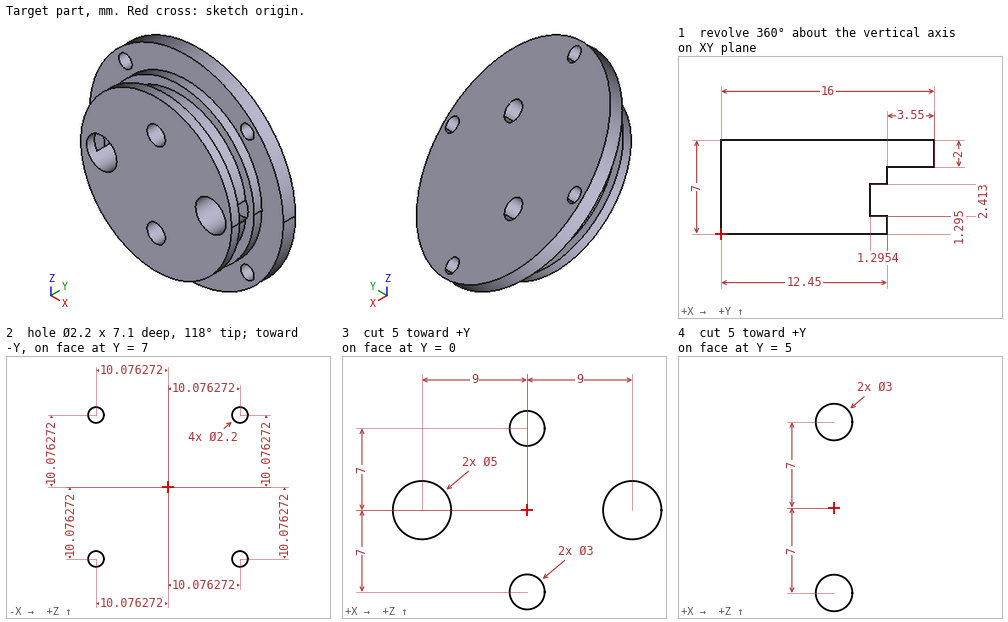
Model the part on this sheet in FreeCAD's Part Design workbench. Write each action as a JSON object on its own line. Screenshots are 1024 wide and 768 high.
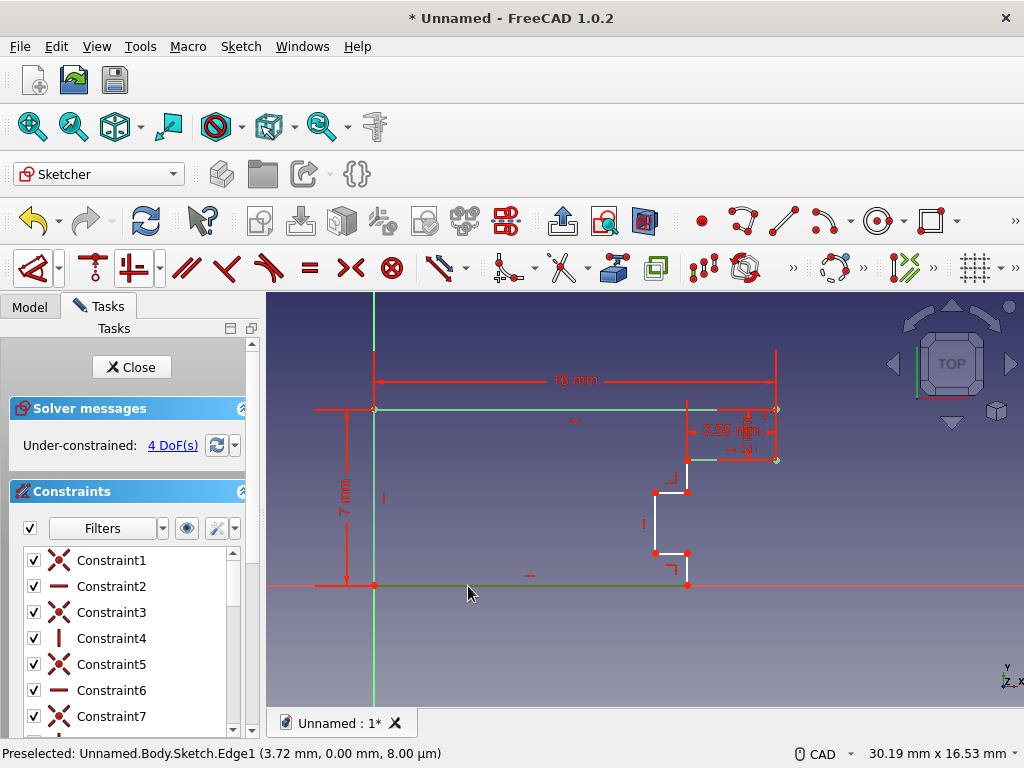
{"action": "left_click", "coordinate": [58, 268]}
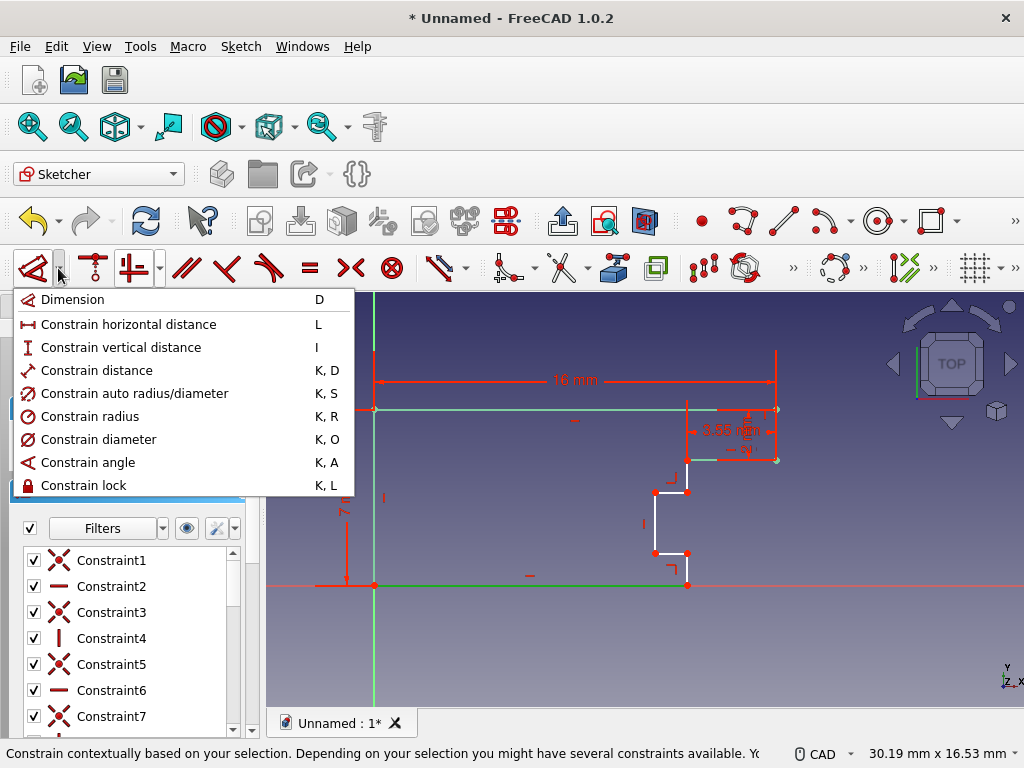
{"action": "left_click", "coordinate": [184, 324]}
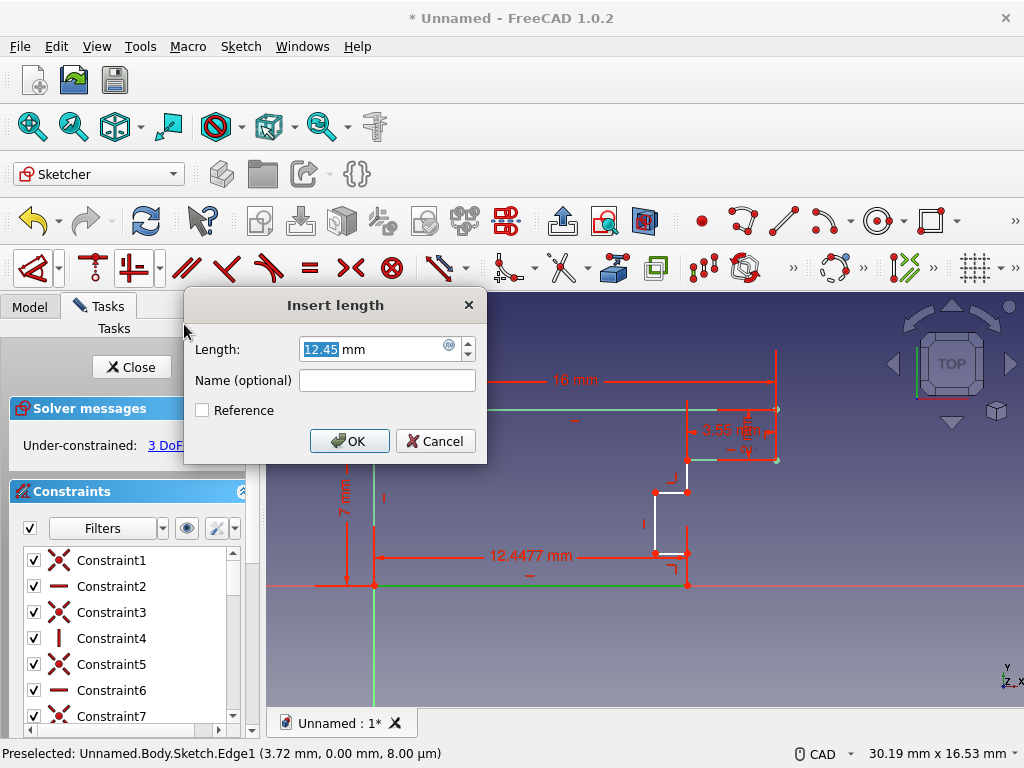
{"action": "type", "text": "12.45"}
{"action": "key", "text": "Return"}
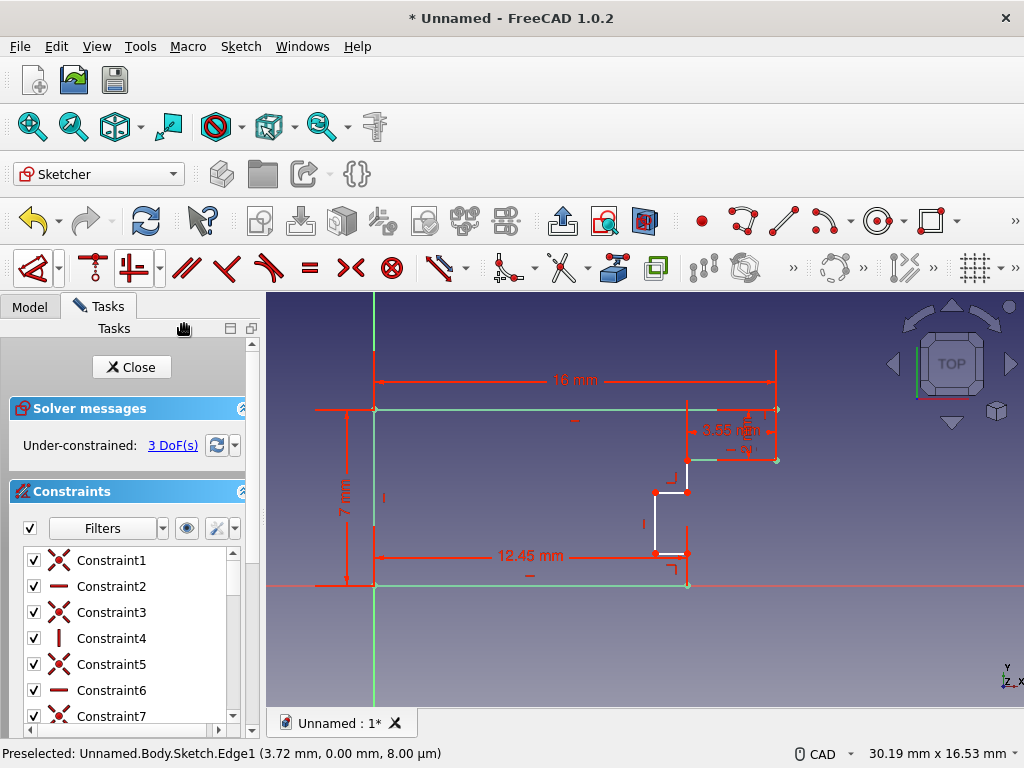
{"action": "scroll", "coordinate": [687, 576], "scroll_direction": "up", "scroll_amount": 2}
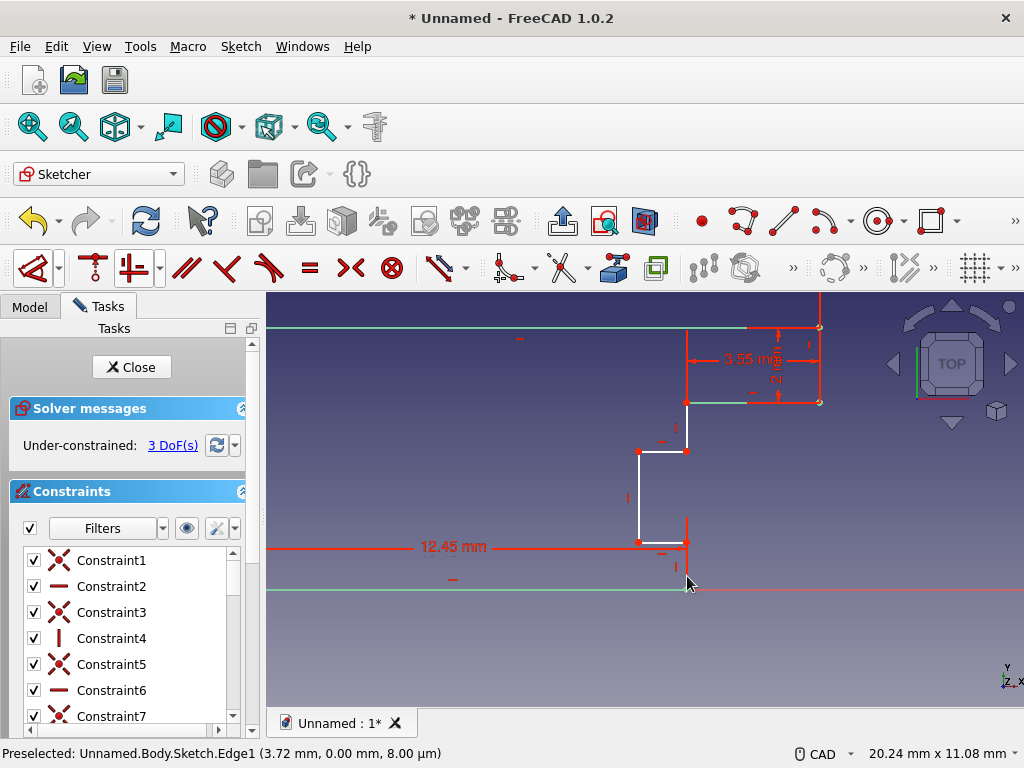
{"action": "left_click", "coordinate": [687, 576]}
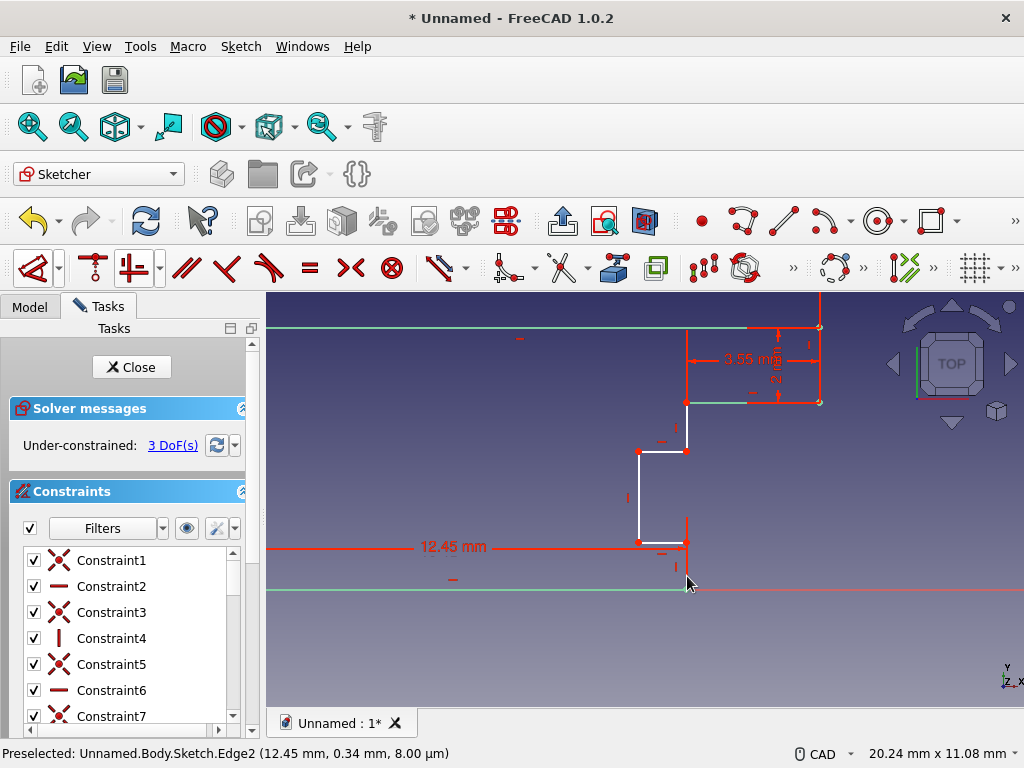
{"action": "key", "text": "i"}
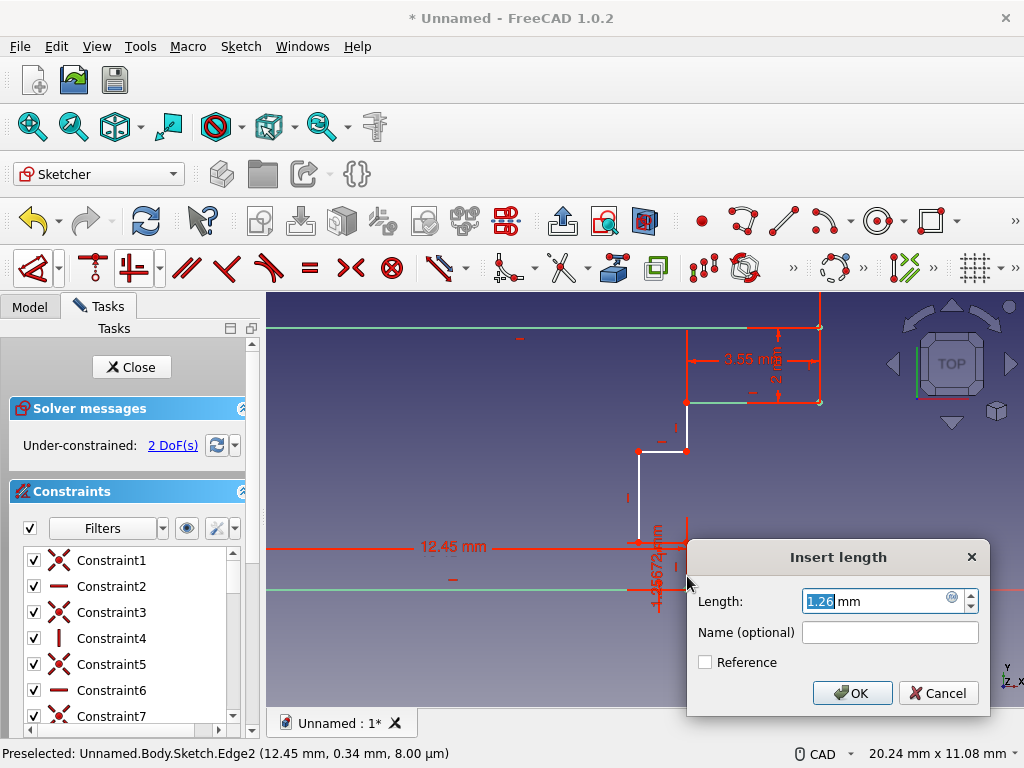
{"action": "type", "text": "1.295"}
{"action": "key", "text": "Return"}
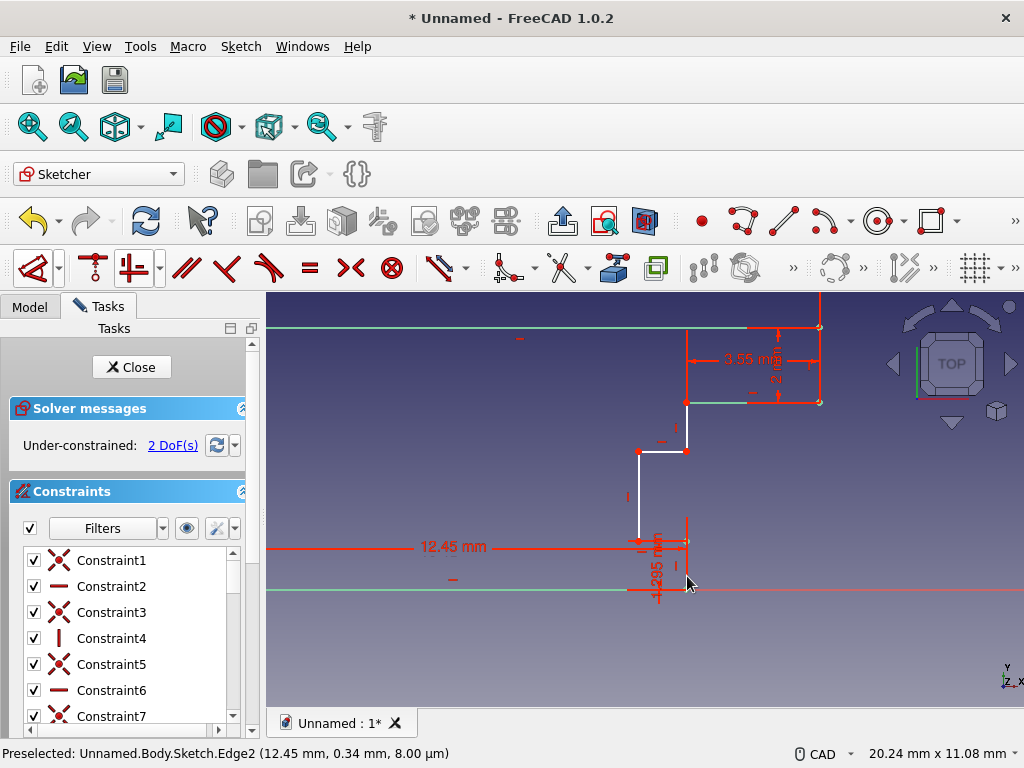
{"action": "left_click", "coordinate": [639, 515]}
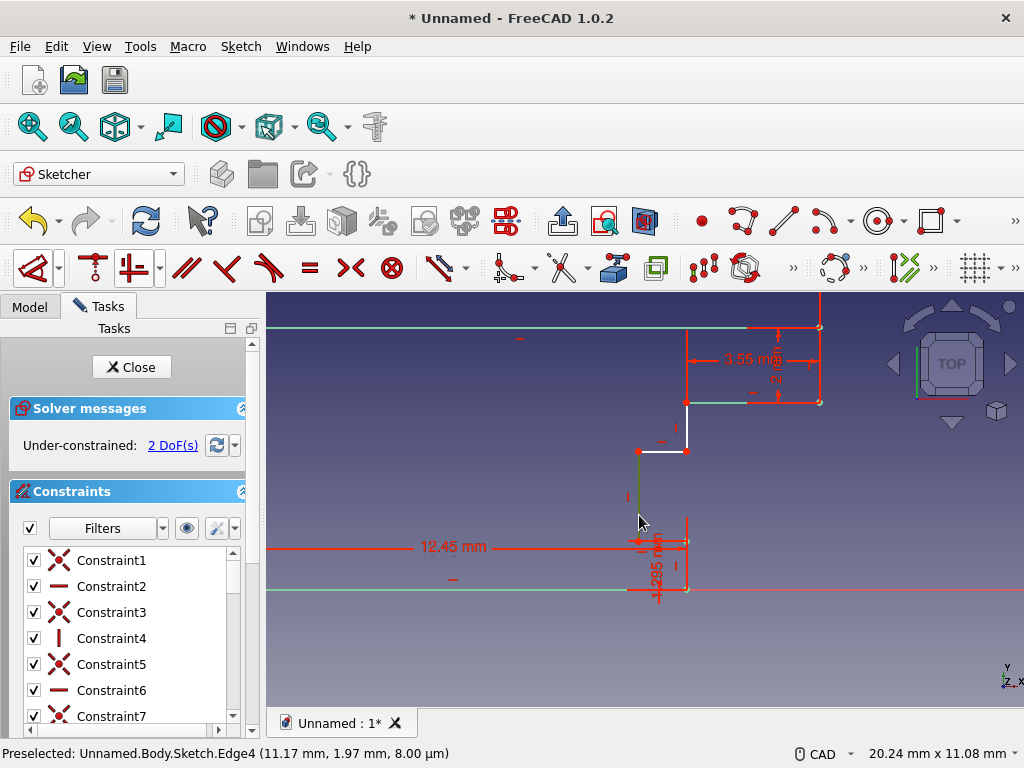
{"action": "key", "text": "i"}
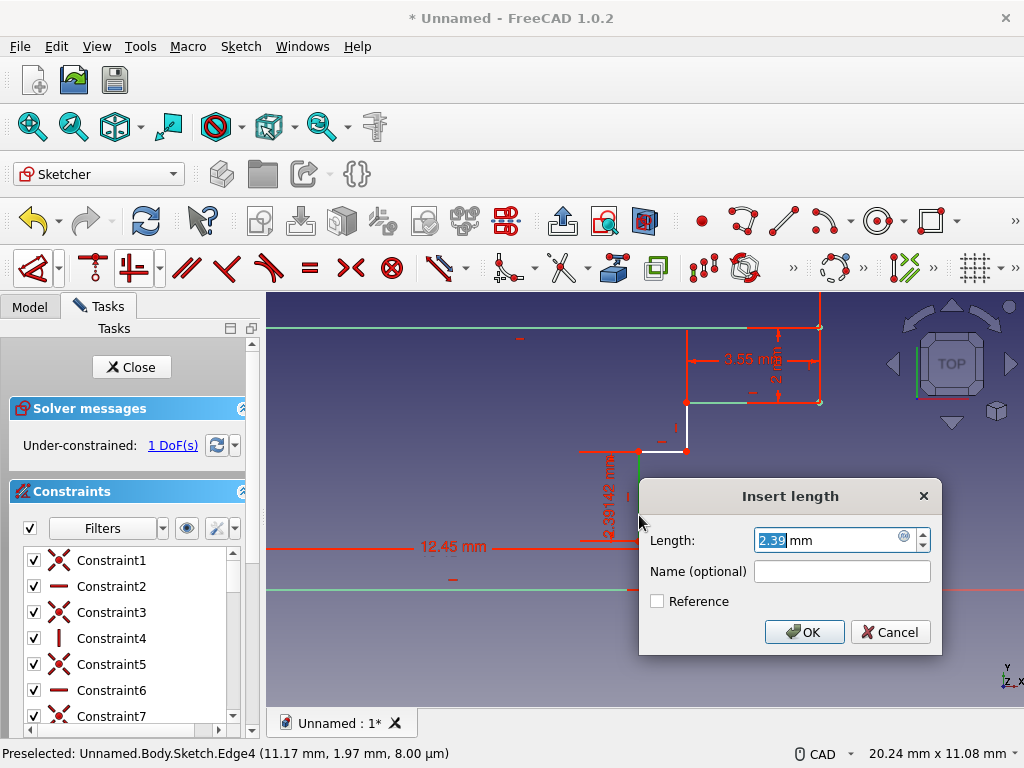
{"action": "type", "text": "2.413"}
{"action": "key", "text": "Return"}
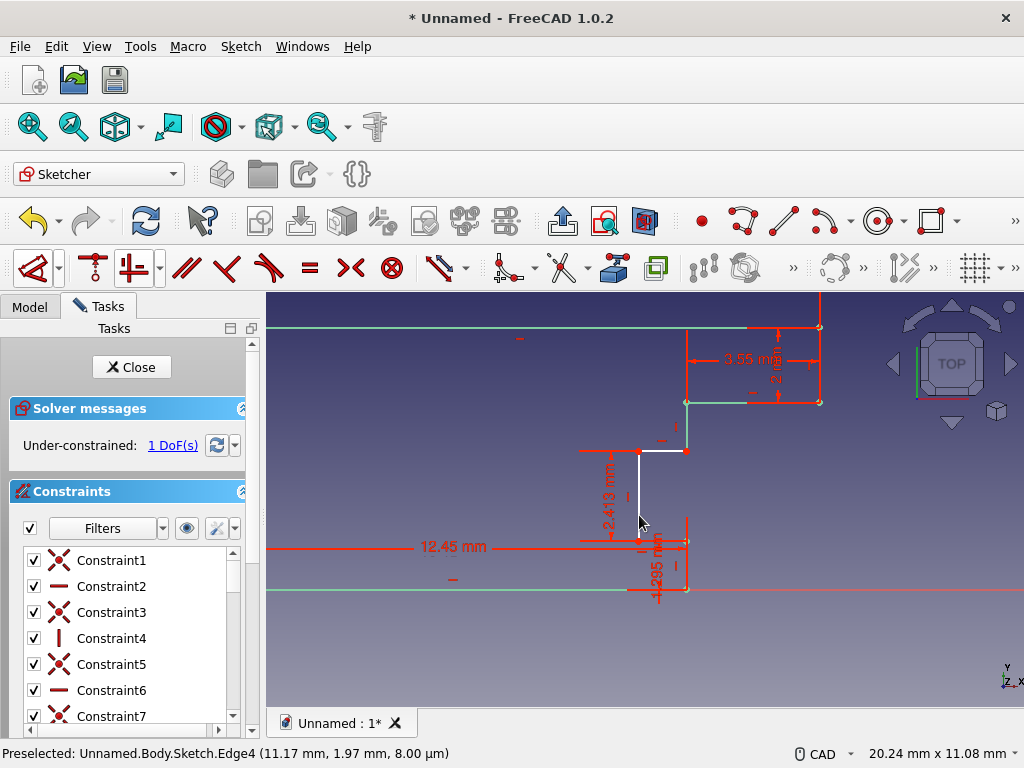
{"action": "left_click", "coordinate": [672, 541]}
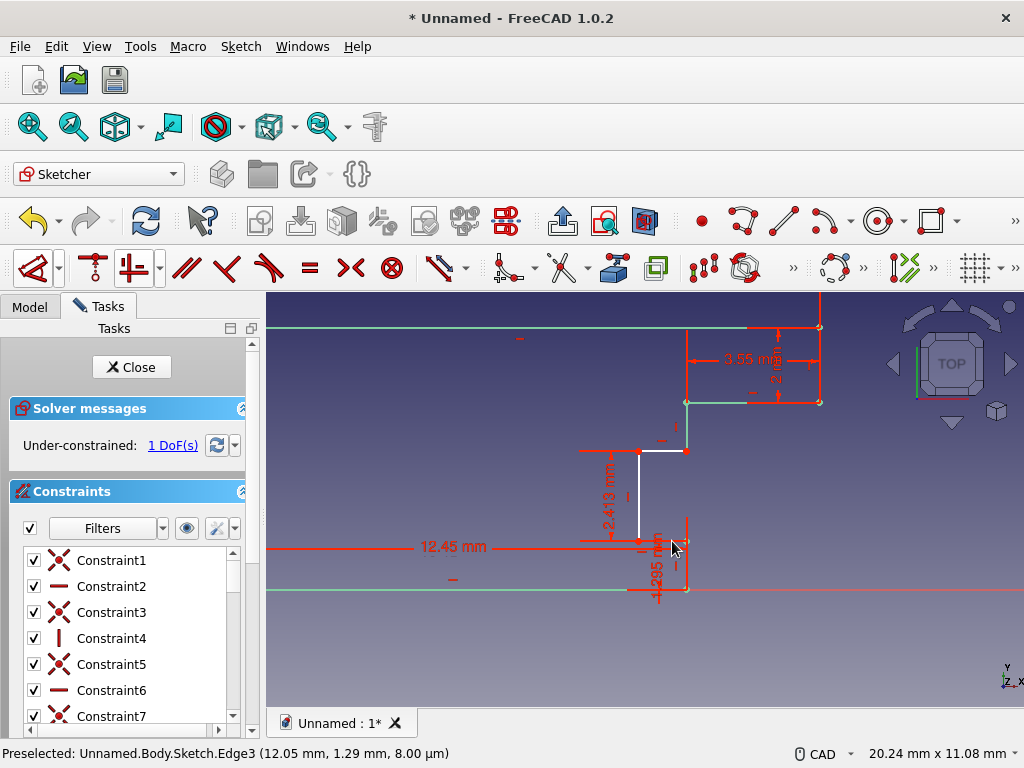
{"action": "left_click", "coordinate": [58, 268]}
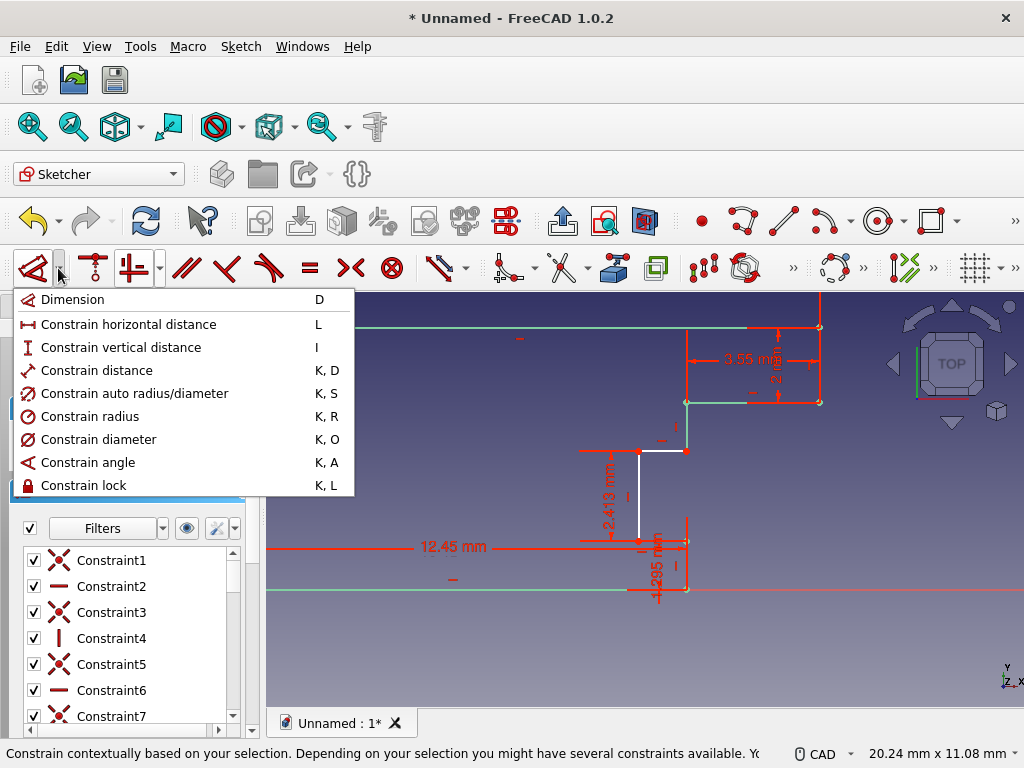
{"action": "left_click", "coordinate": [184, 324]}